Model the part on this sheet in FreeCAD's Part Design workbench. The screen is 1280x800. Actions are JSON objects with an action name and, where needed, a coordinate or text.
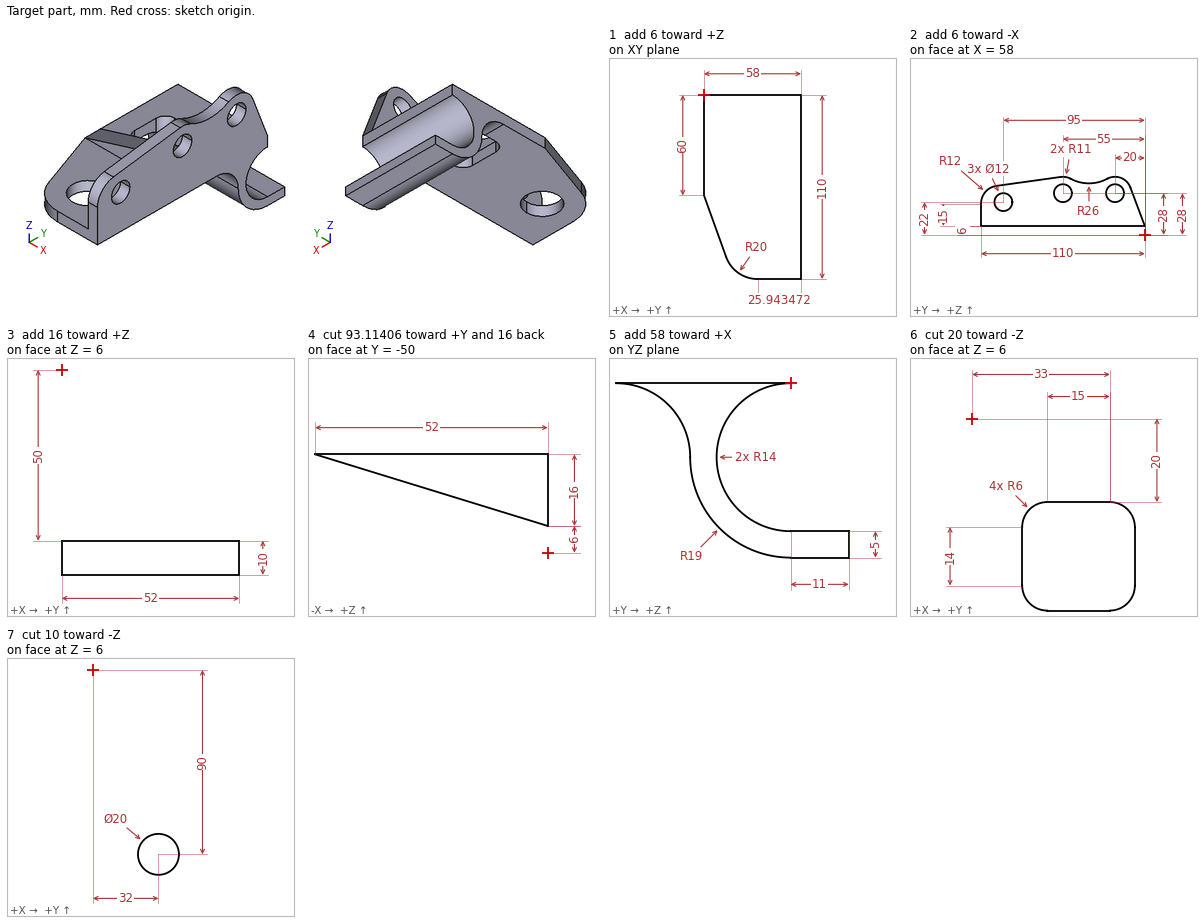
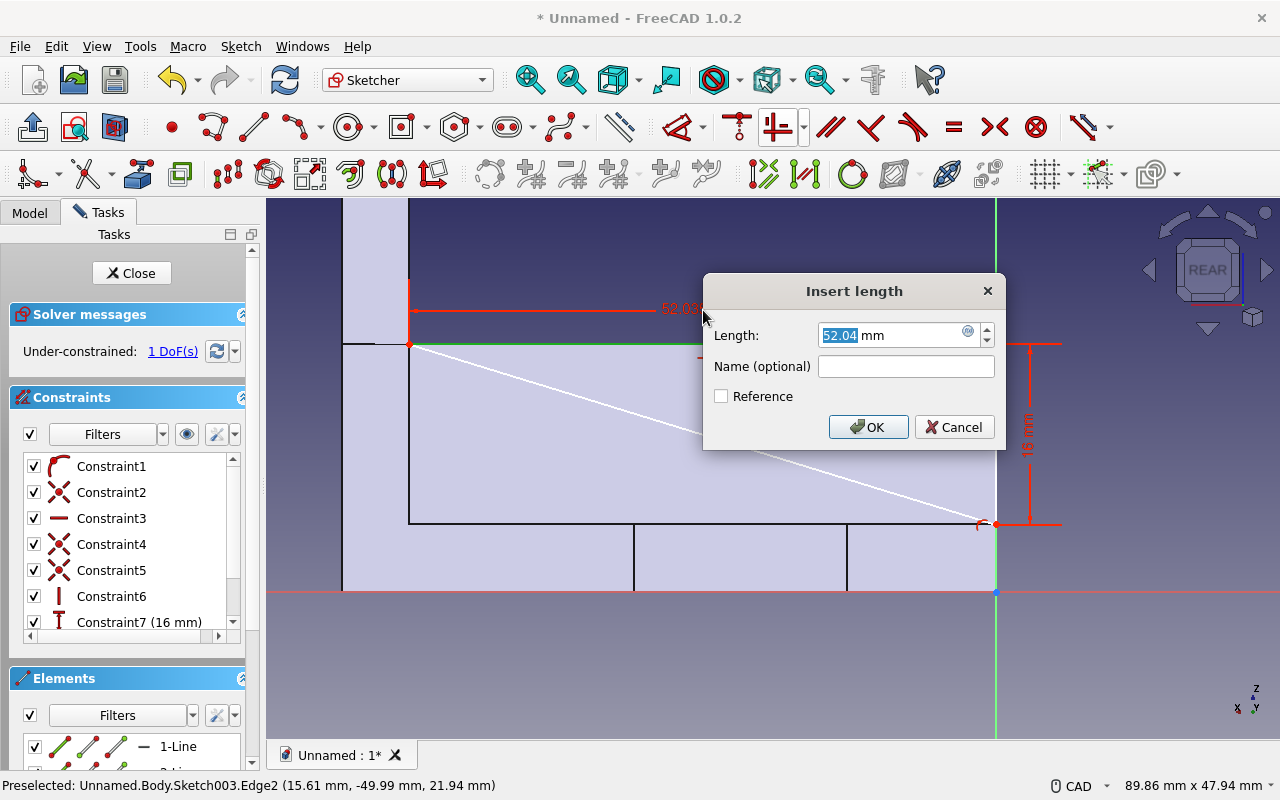
{"action": "type", "text": "52"}
{"action": "key", "text": "Return"}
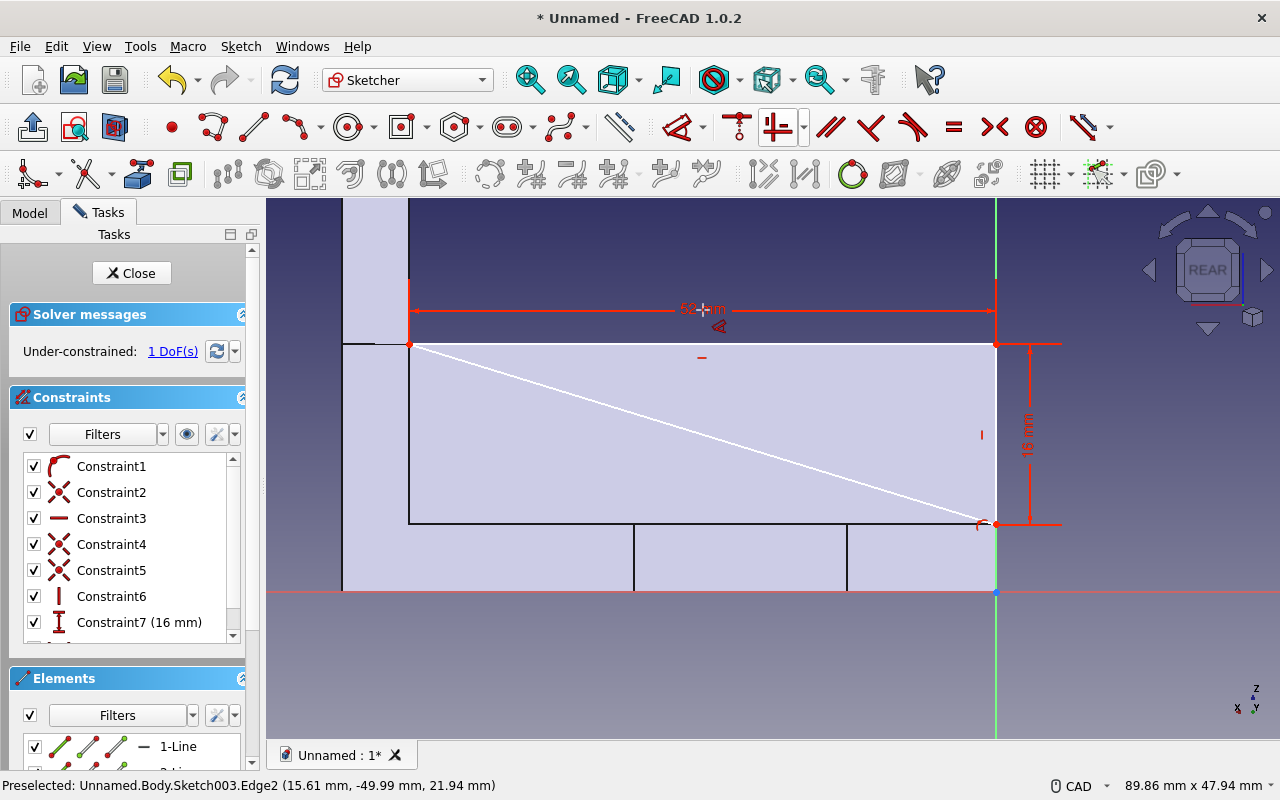
{"action": "left_click", "coordinate": [996, 525]}
{"action": "left_click", "coordinate": [1030, 559]}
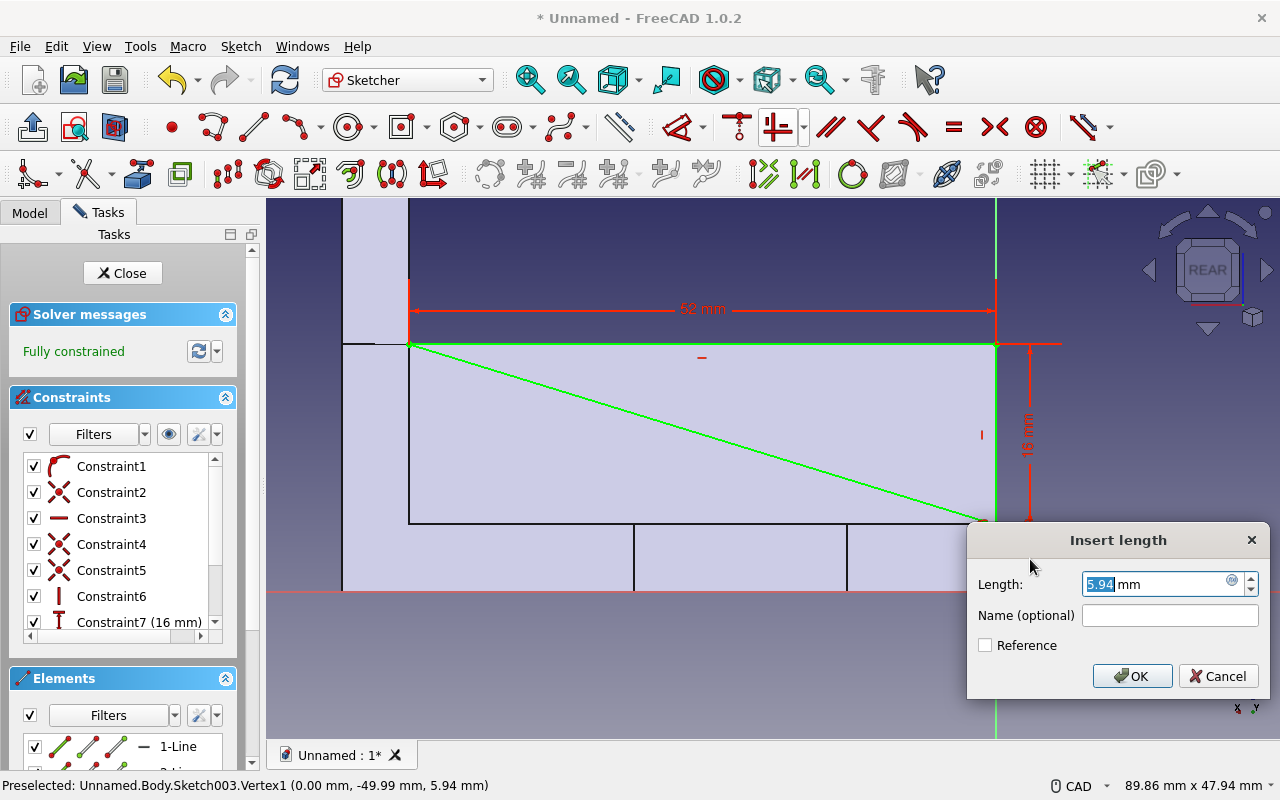
{"action": "type", "text": "6"}
{"action": "key", "text": "Return"}
{"action": "key", "text": "Escape"}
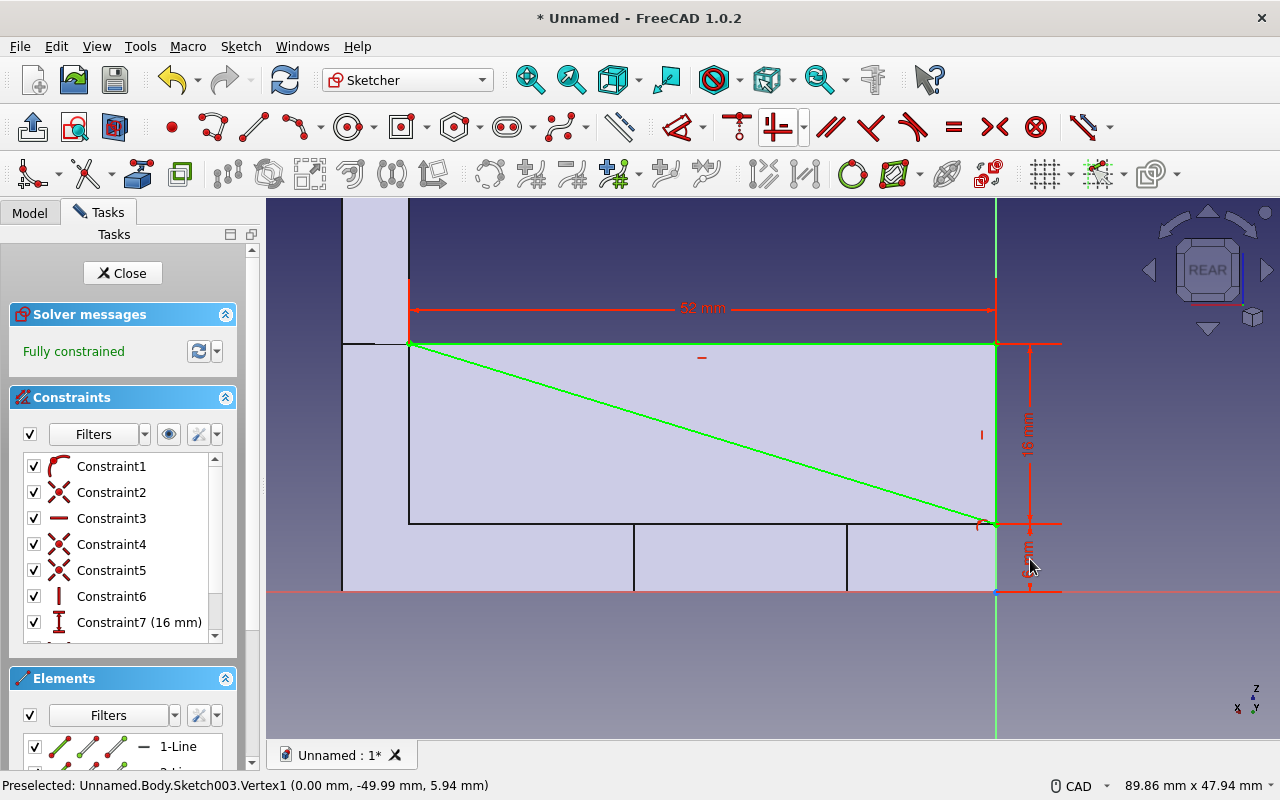
{"action": "left_click", "coordinate": [123, 273]}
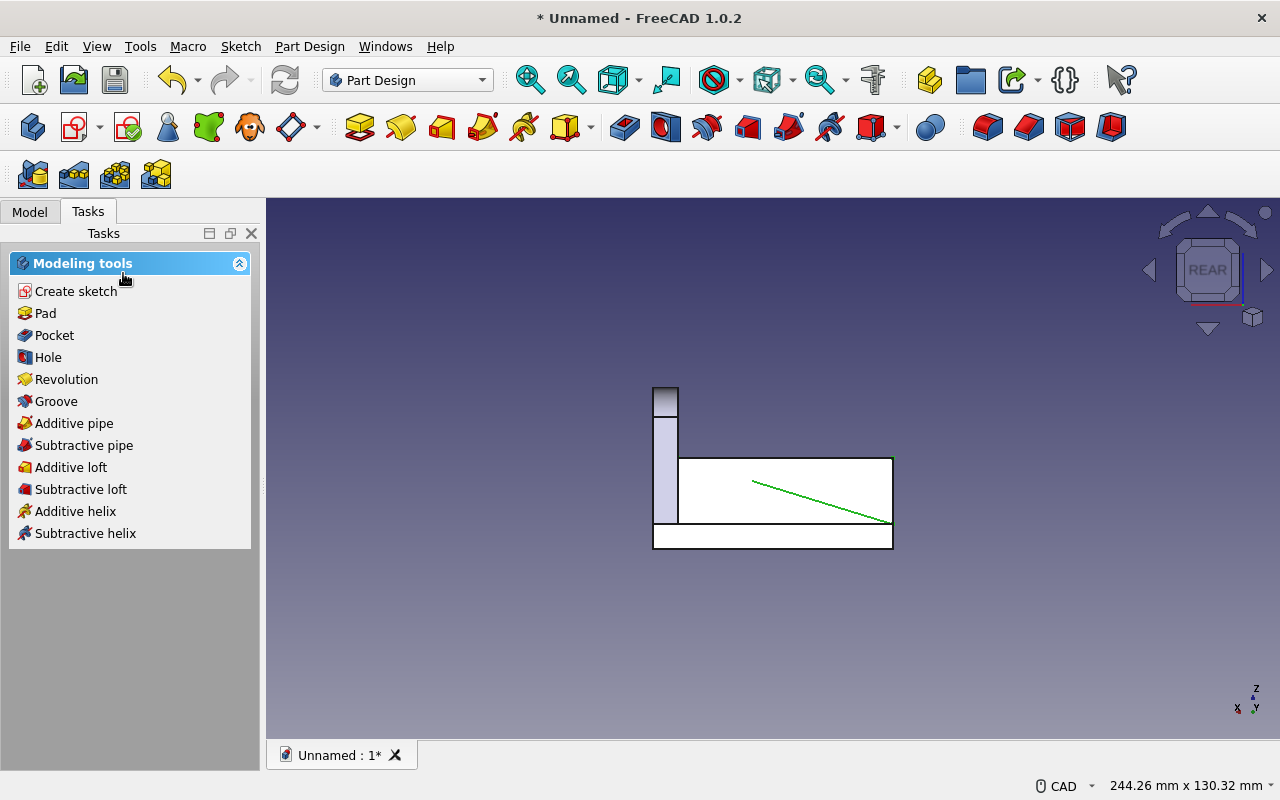
{"action": "left_click", "coordinate": [625, 128]}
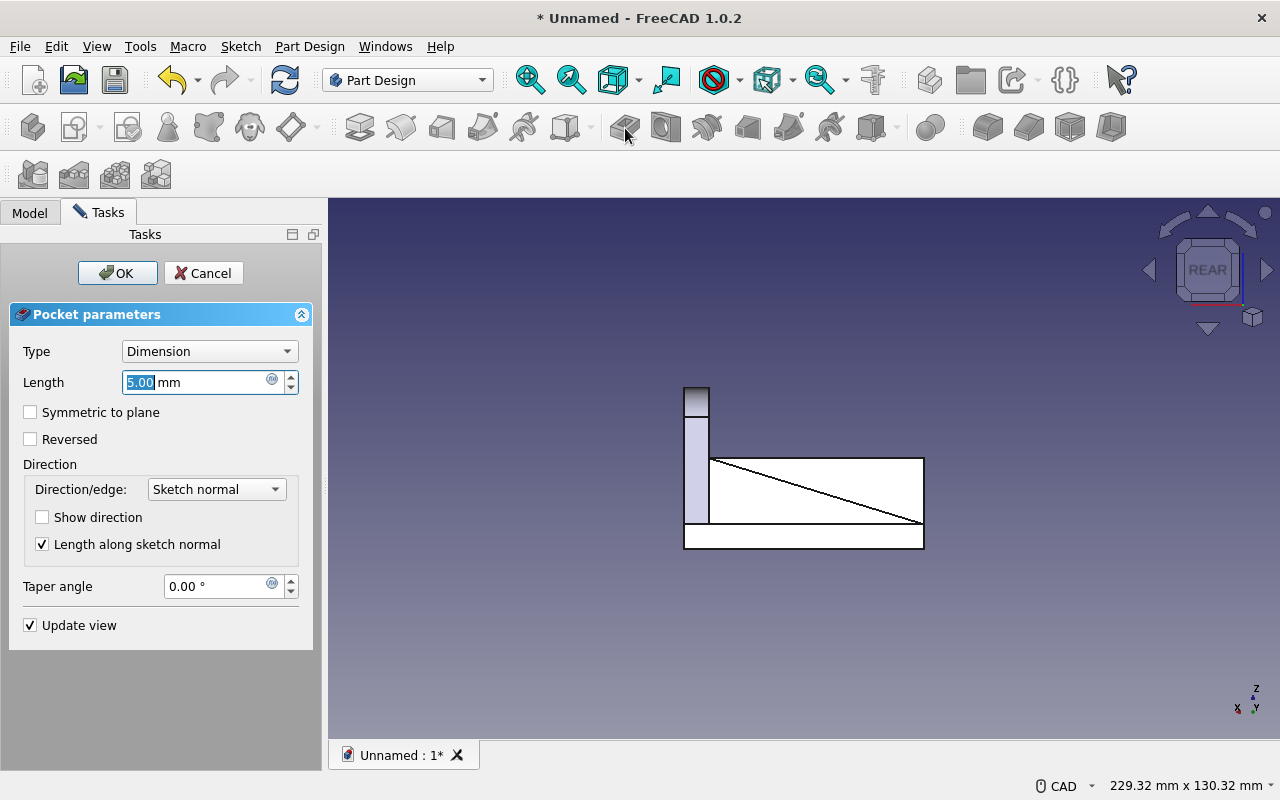
{"action": "left_click", "coordinate": [210, 352]}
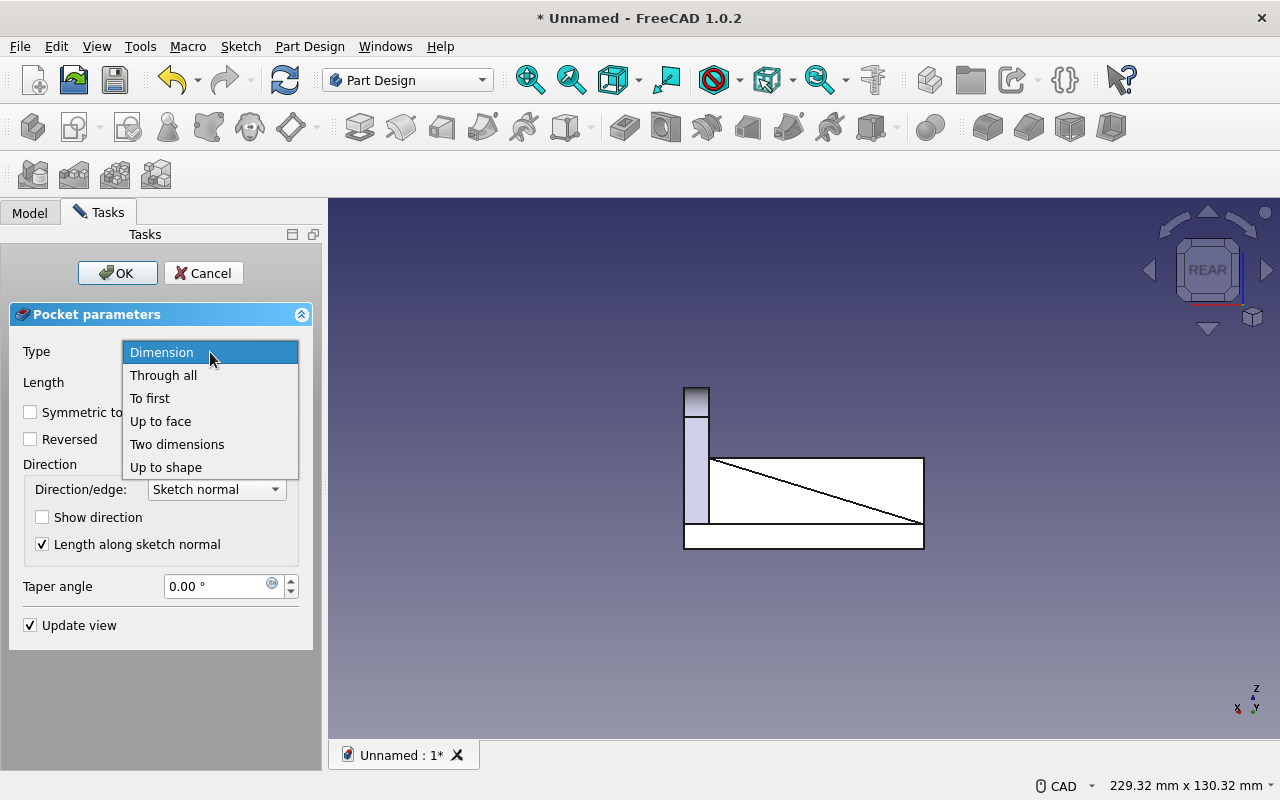
{"action": "left_click", "coordinate": [208, 444]}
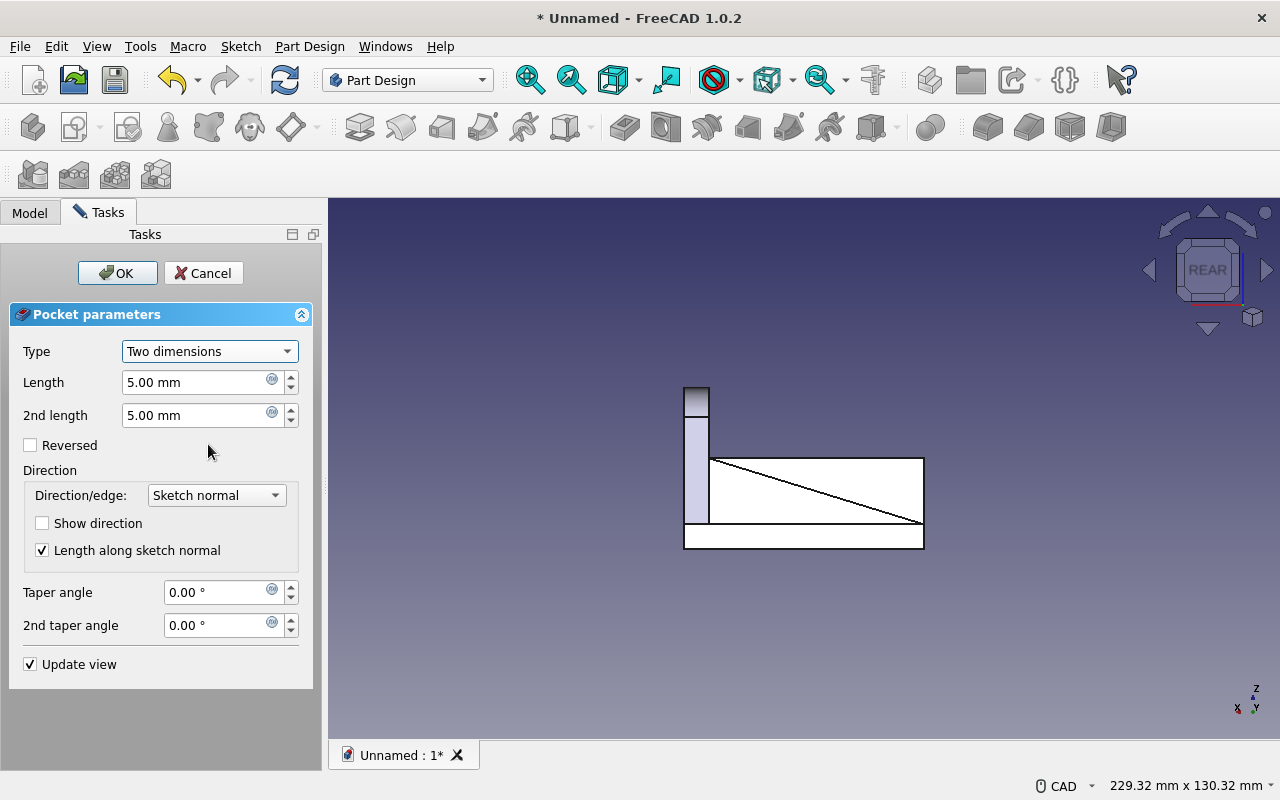
{"action": "triple_click", "coordinate": [204, 382]}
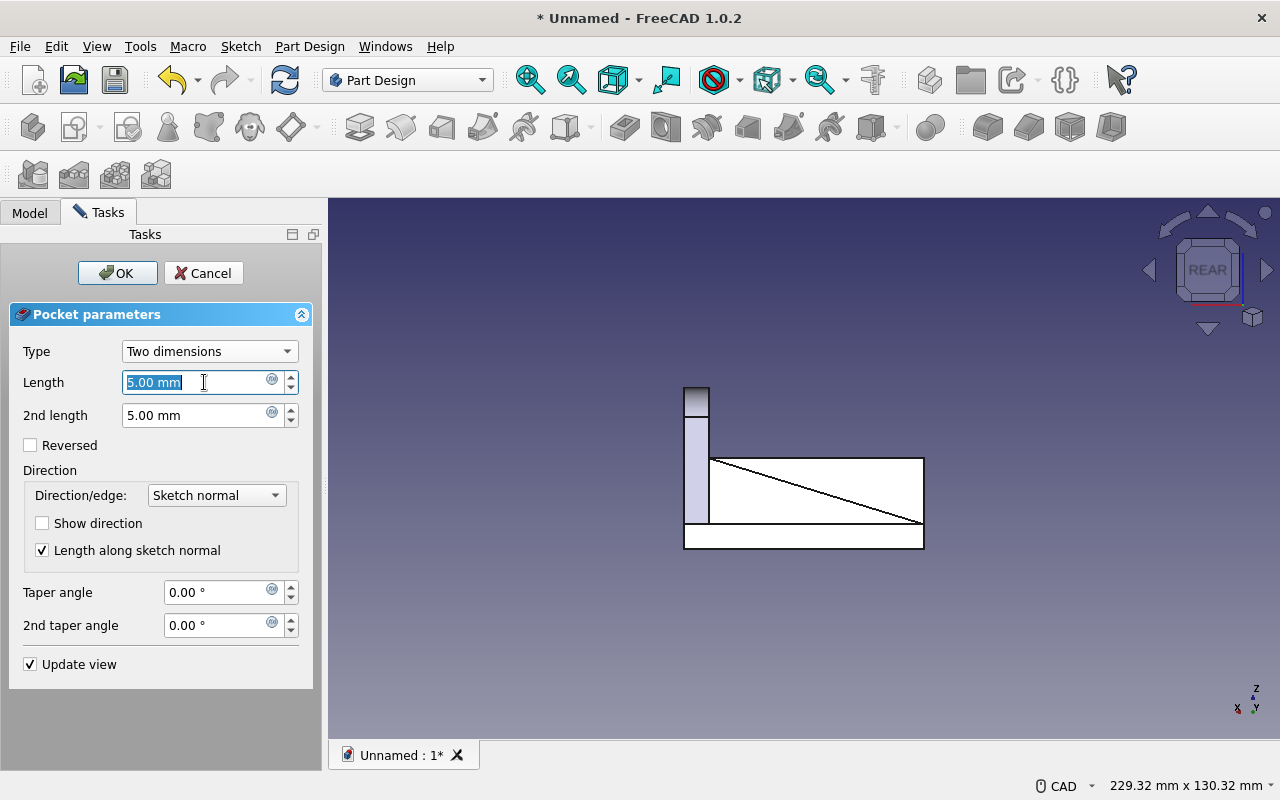
{"action": "type", "text": "93.11406"}
{"action": "key", "text": "Tab"}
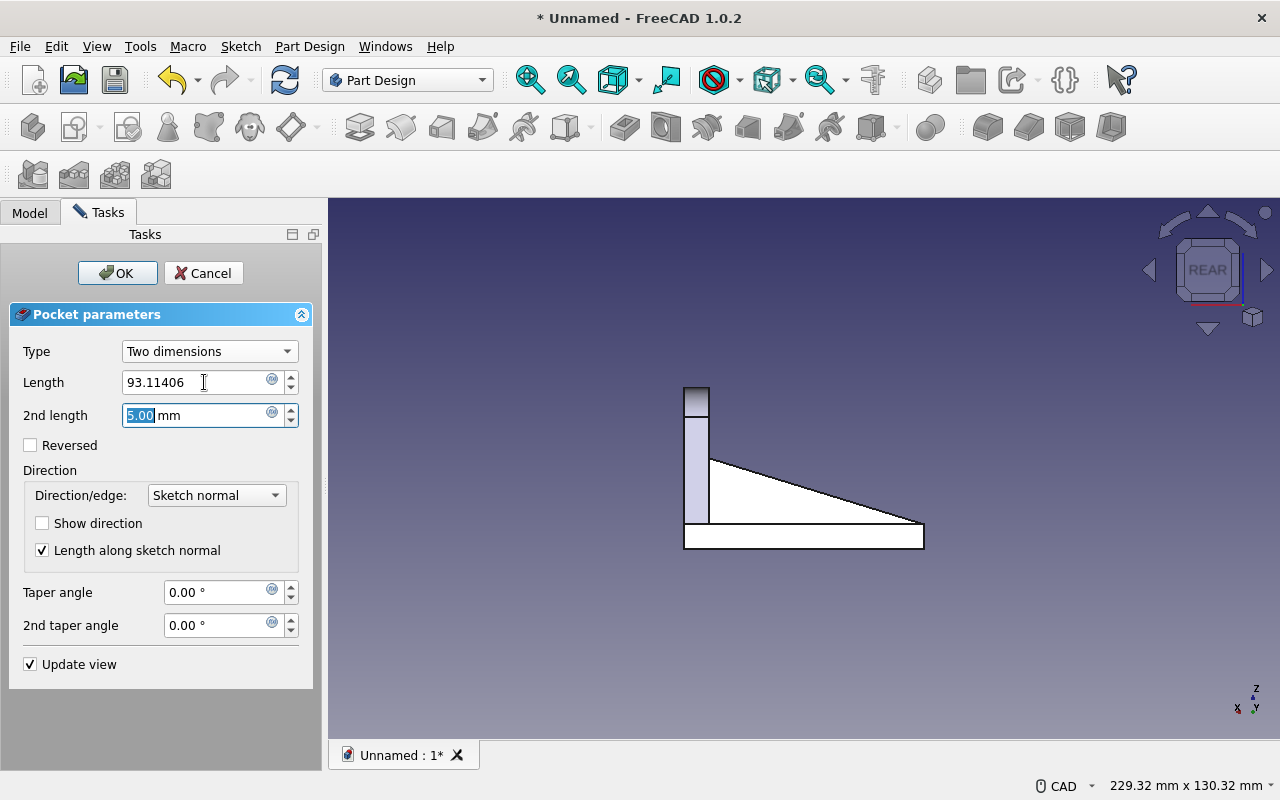
{"action": "type", "text": "16"}
{"action": "key", "text": "Tab"}